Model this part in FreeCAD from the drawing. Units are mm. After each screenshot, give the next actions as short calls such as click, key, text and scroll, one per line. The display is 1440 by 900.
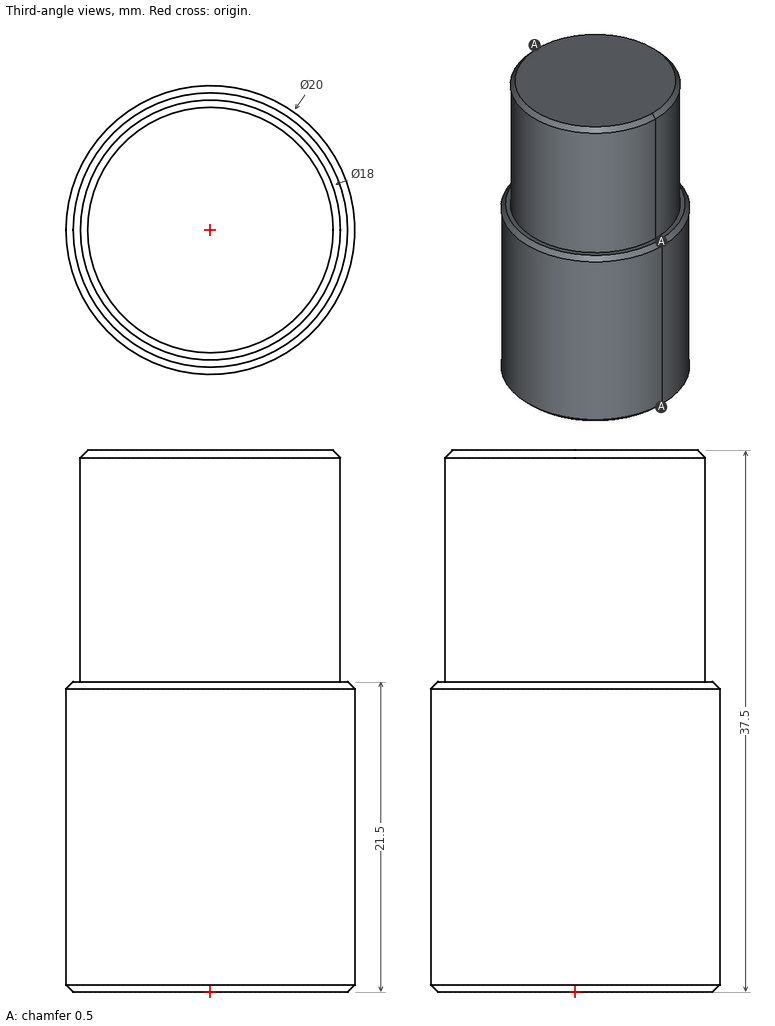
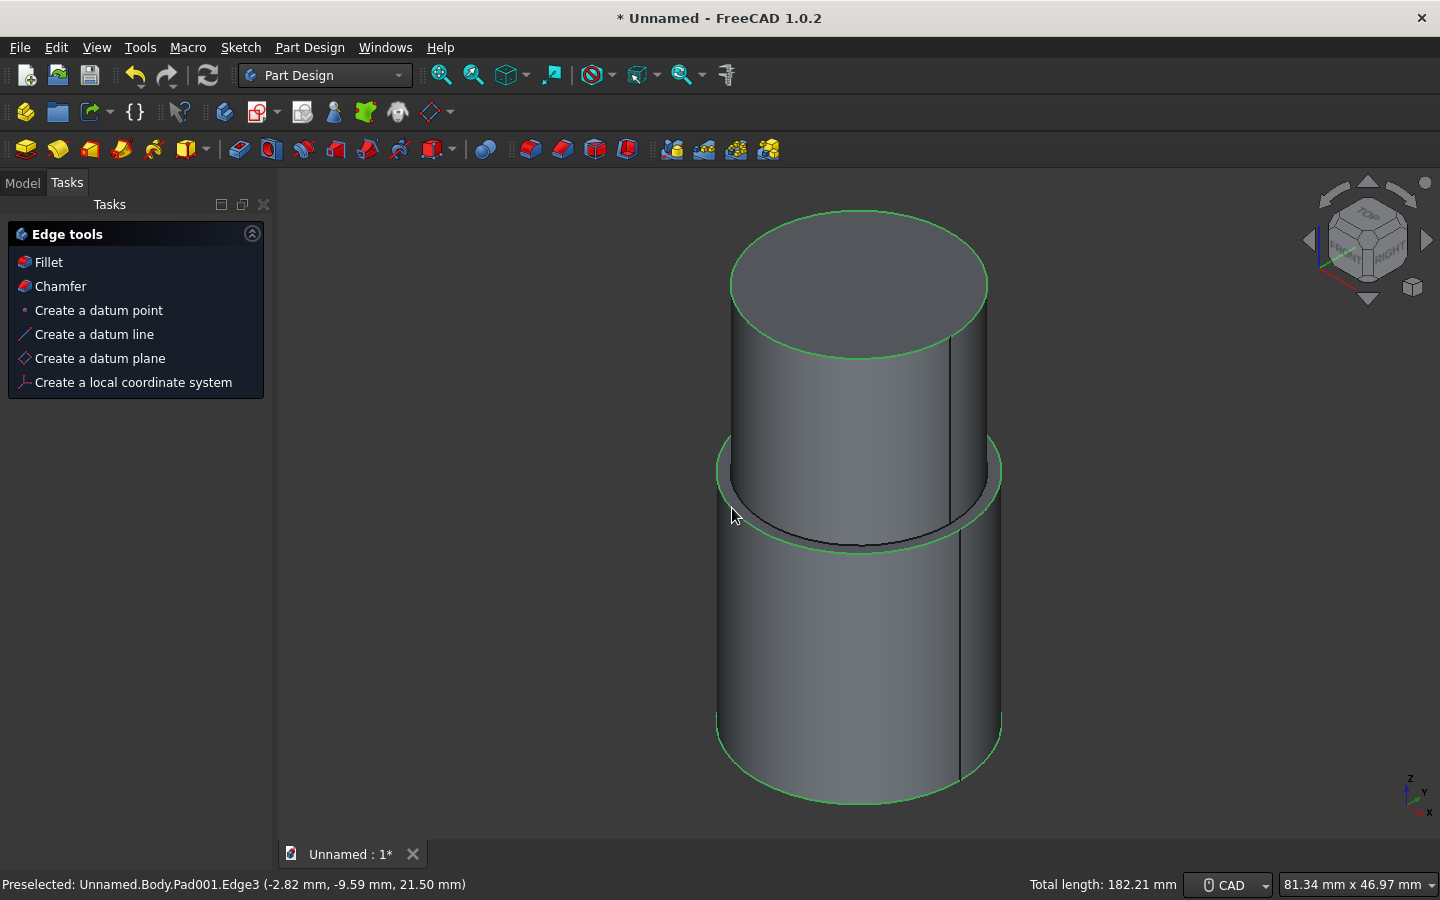
click(564, 150)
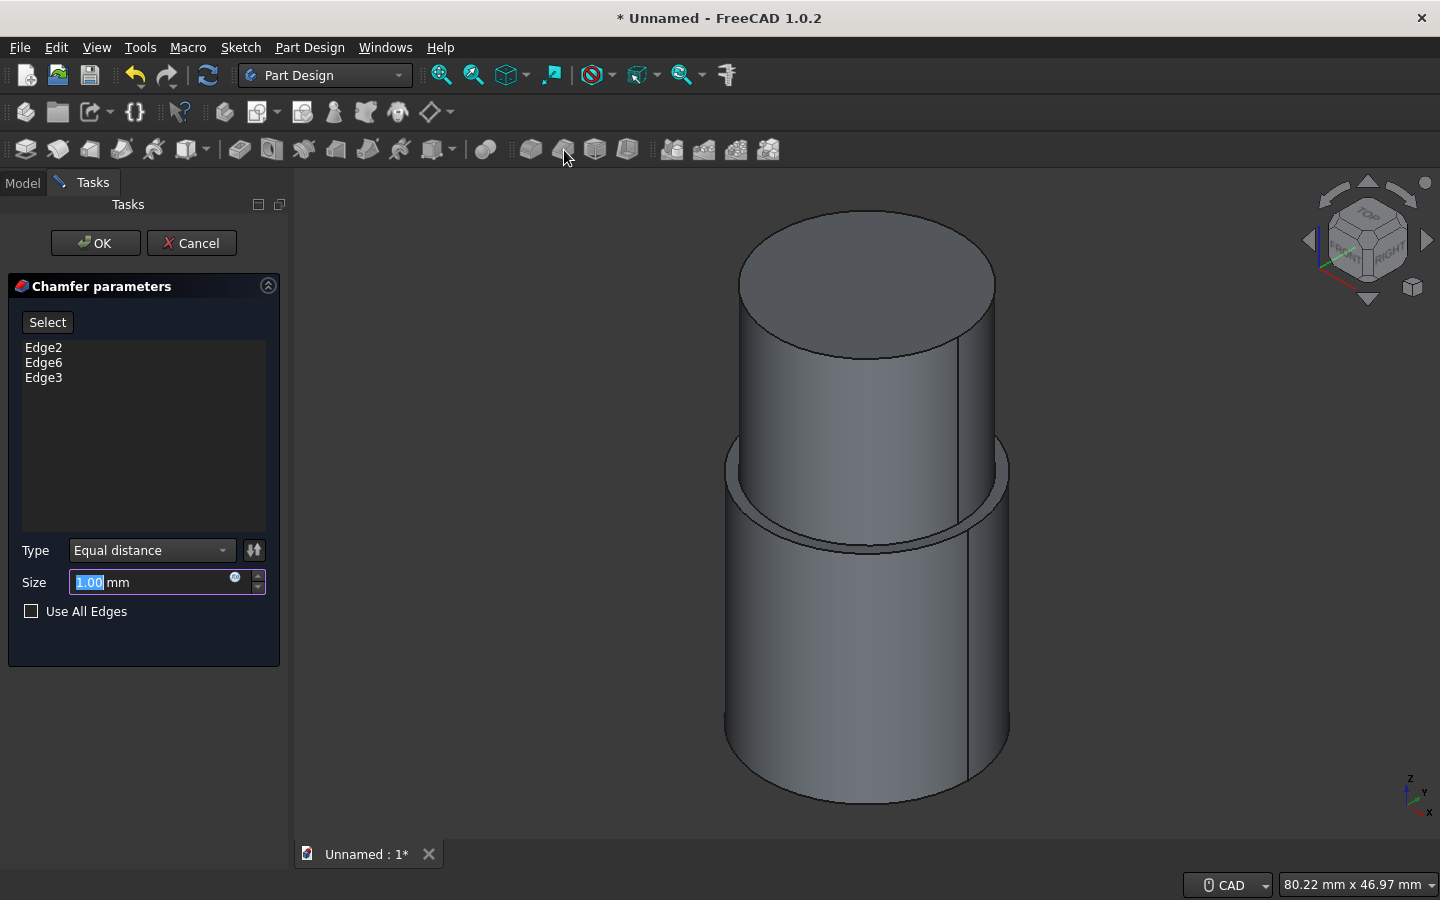
text(0.5)
key(Tab)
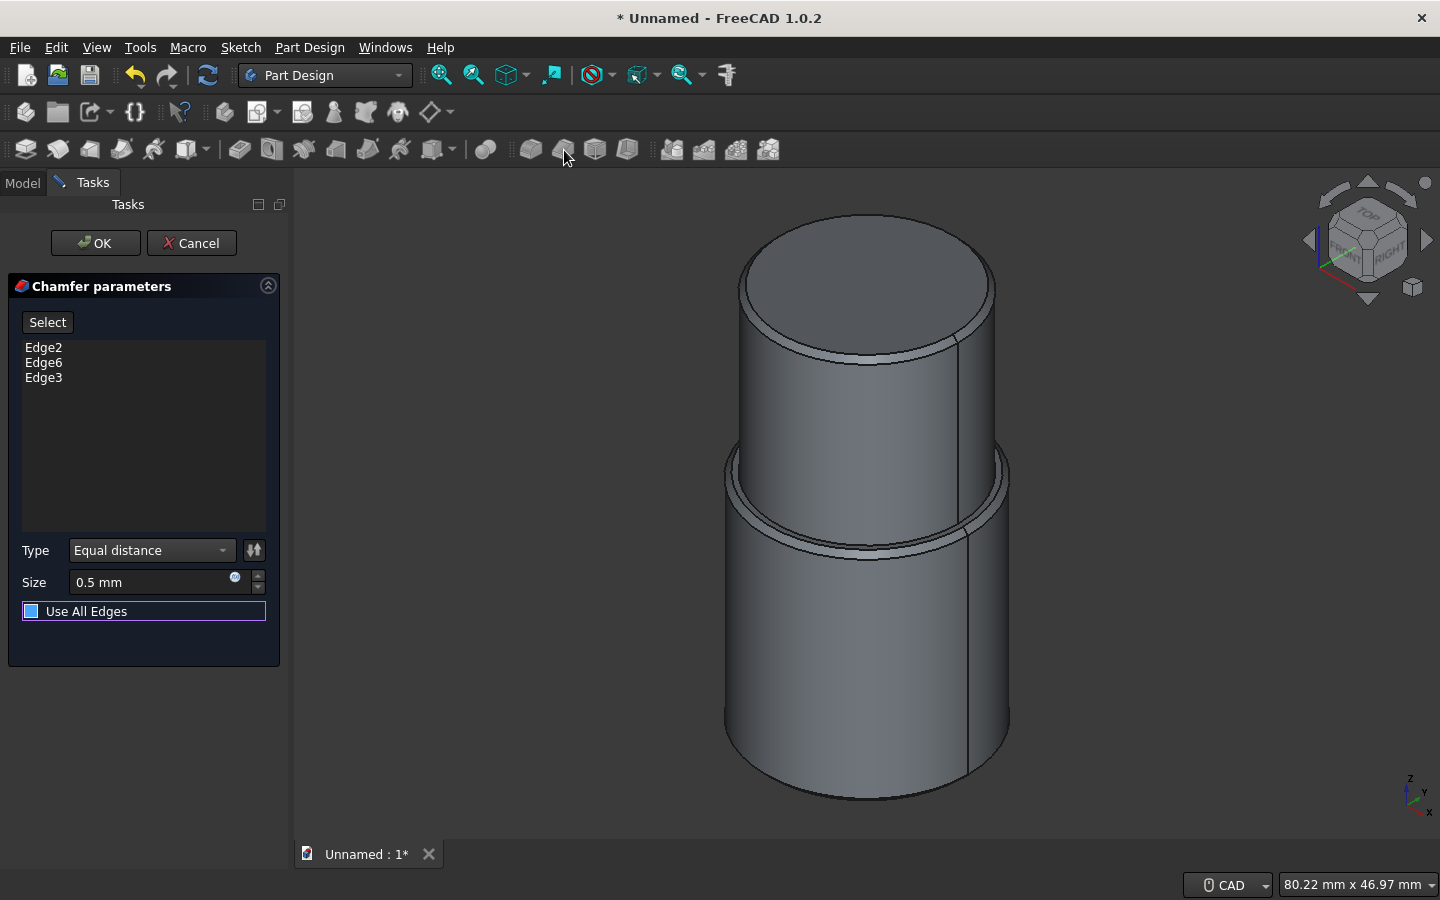
click(96, 243)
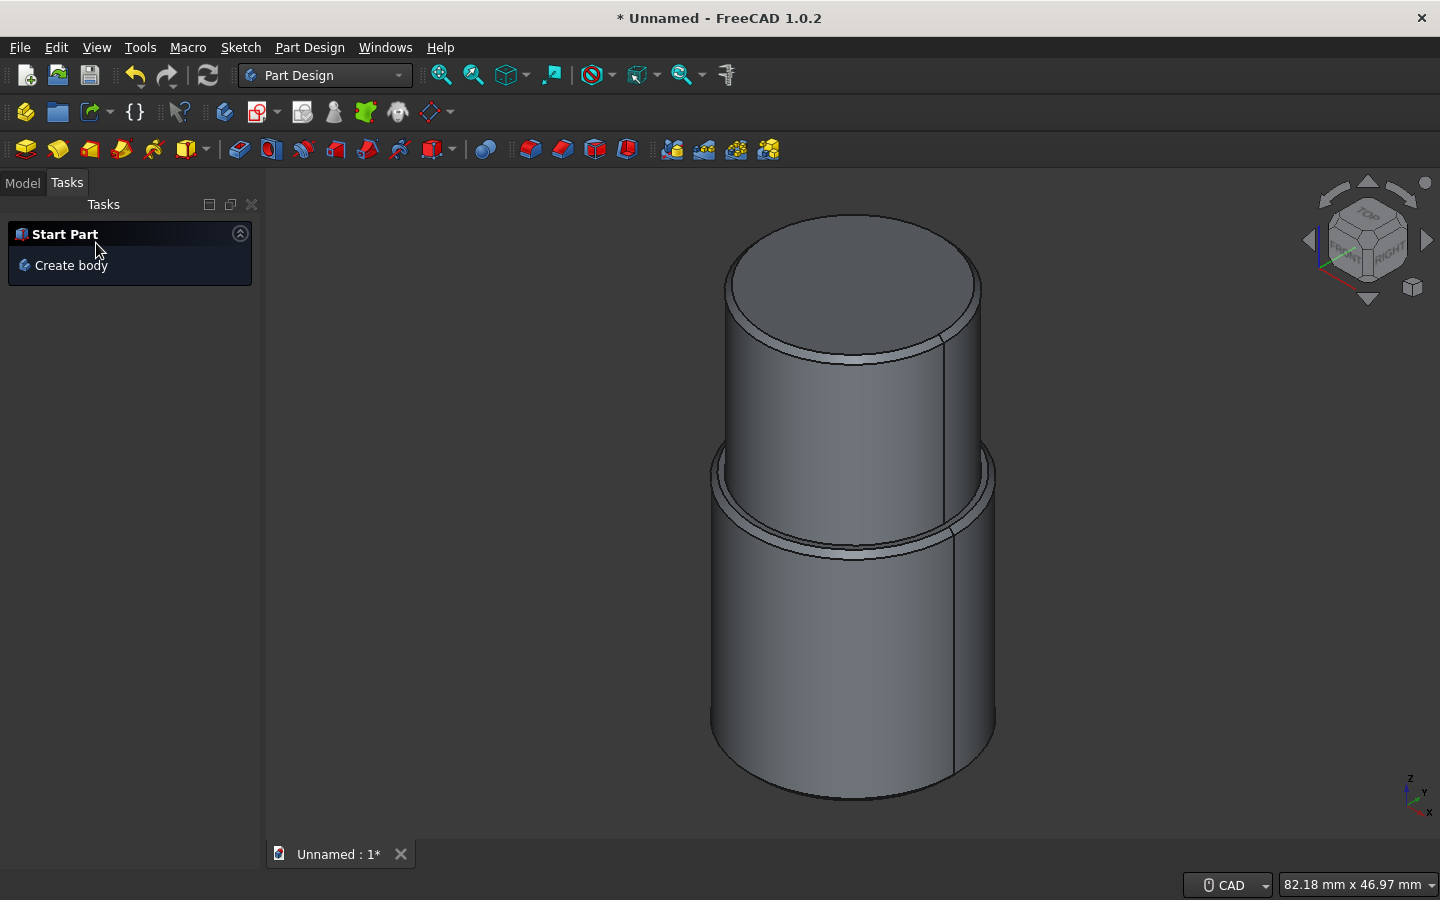
click(442, 76)